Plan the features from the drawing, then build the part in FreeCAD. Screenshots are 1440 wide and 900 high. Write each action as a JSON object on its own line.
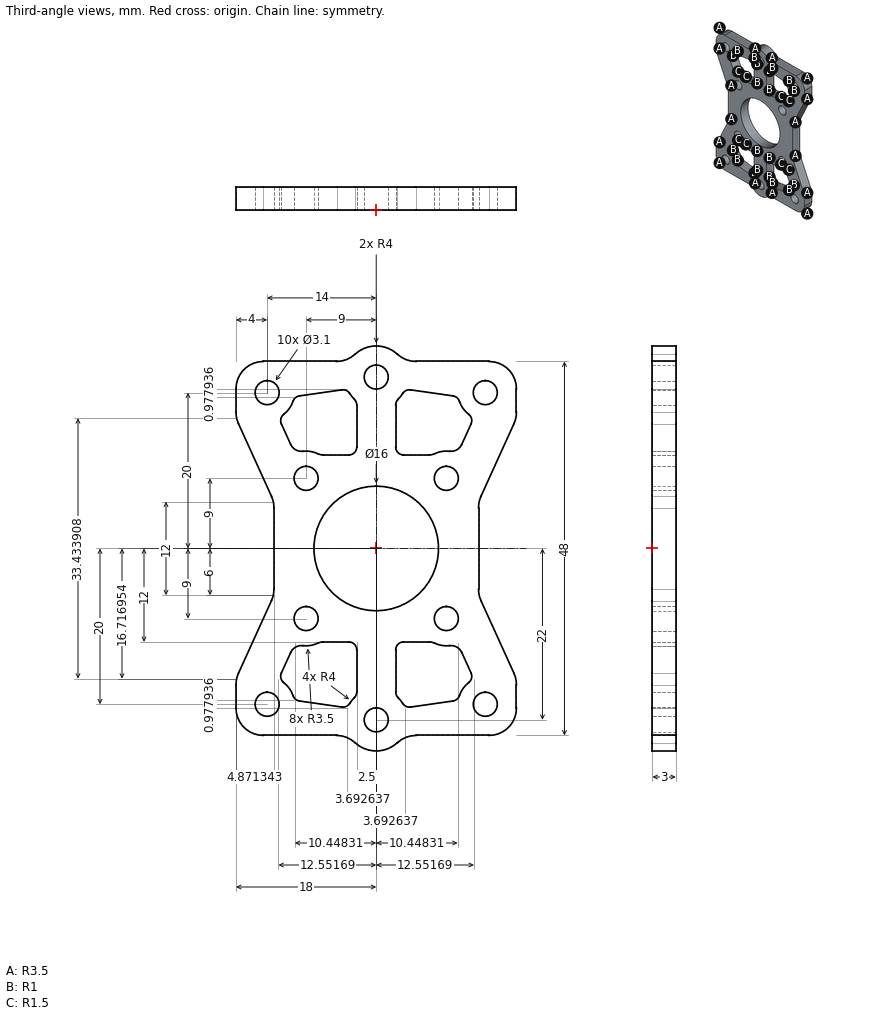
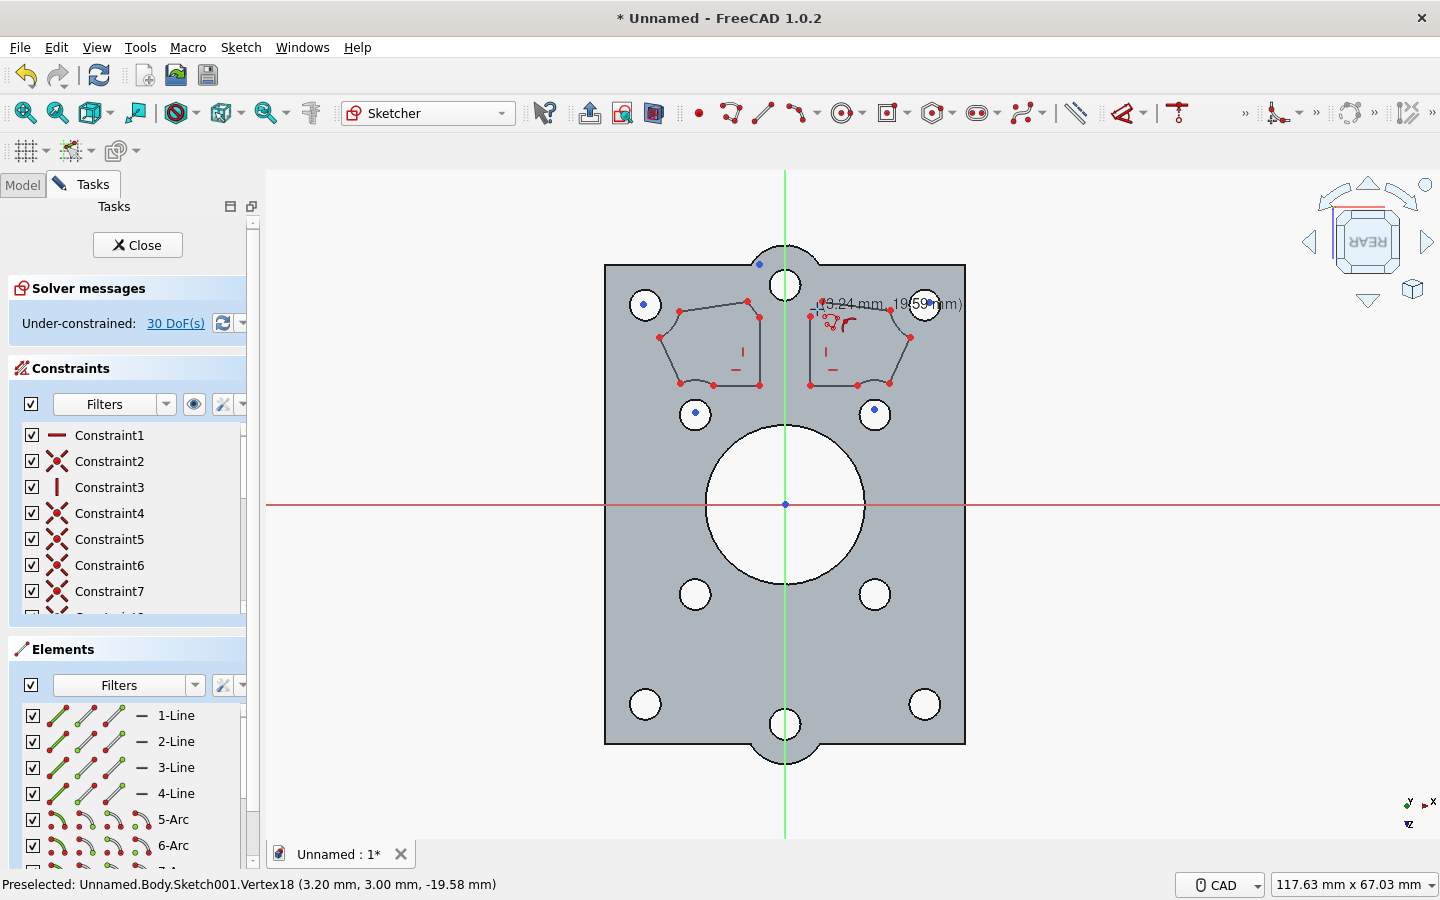
{"action": "left_click", "coordinate": [654, 445]}
{"action": "left_click", "coordinate": [605, 338]}
{"action": "left_click", "coordinate": [605, 672]}
{"action": "left_click", "coordinate": [654, 565]}
{"action": "left_click", "coordinate": [654, 446]}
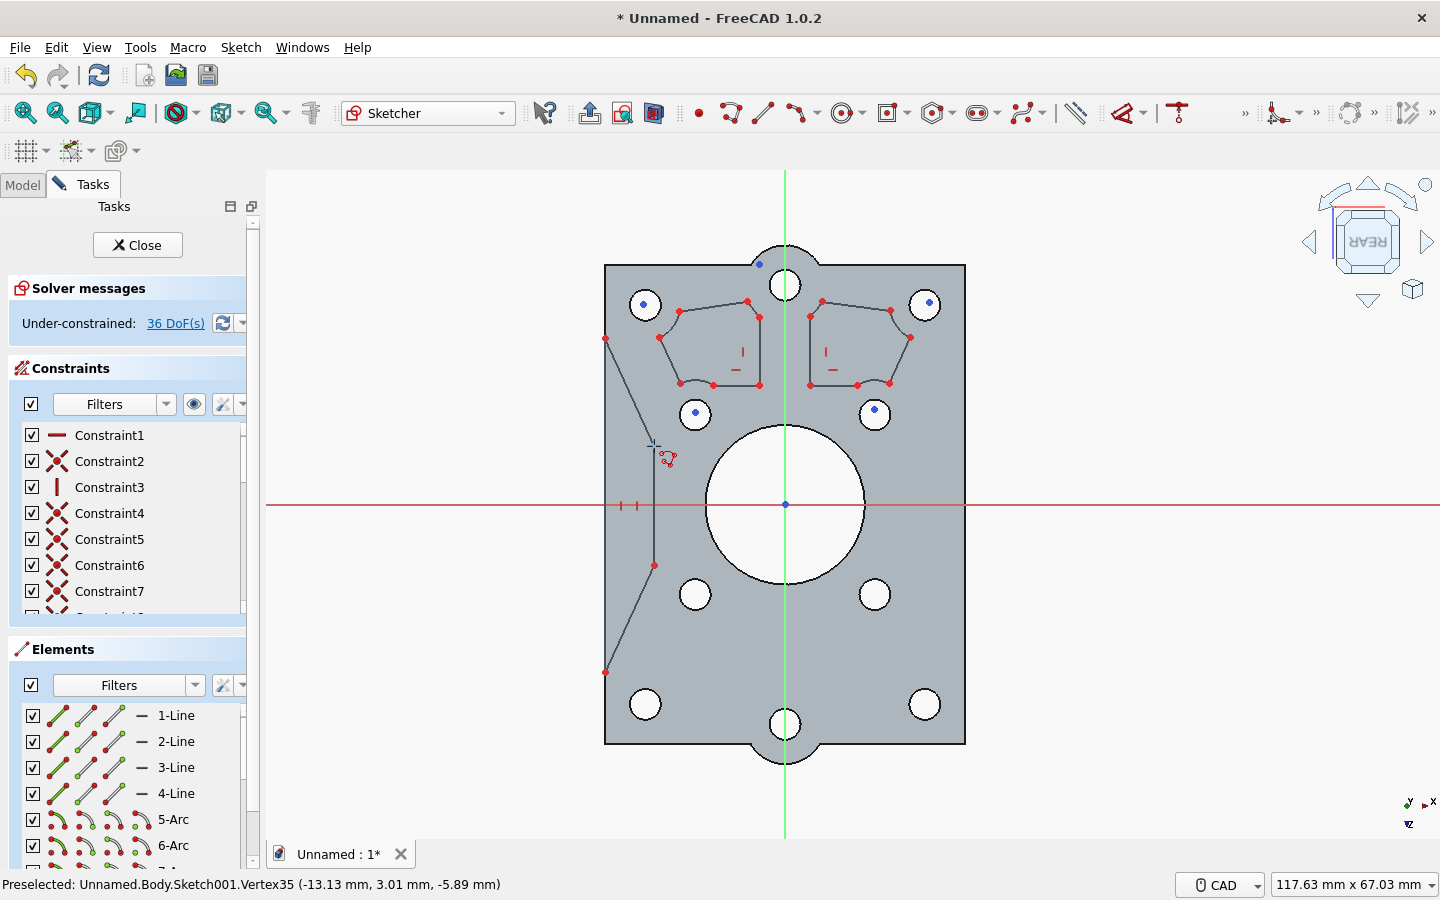
{"action": "left_click", "coordinate": [916, 445]}
{"action": "left_click", "coordinate": [916, 565]}
{"action": "left_click", "coordinate": [965, 672]}
{"action": "left_click", "coordinate": [965, 338]}
{"action": "left_click", "coordinate": [916, 446]}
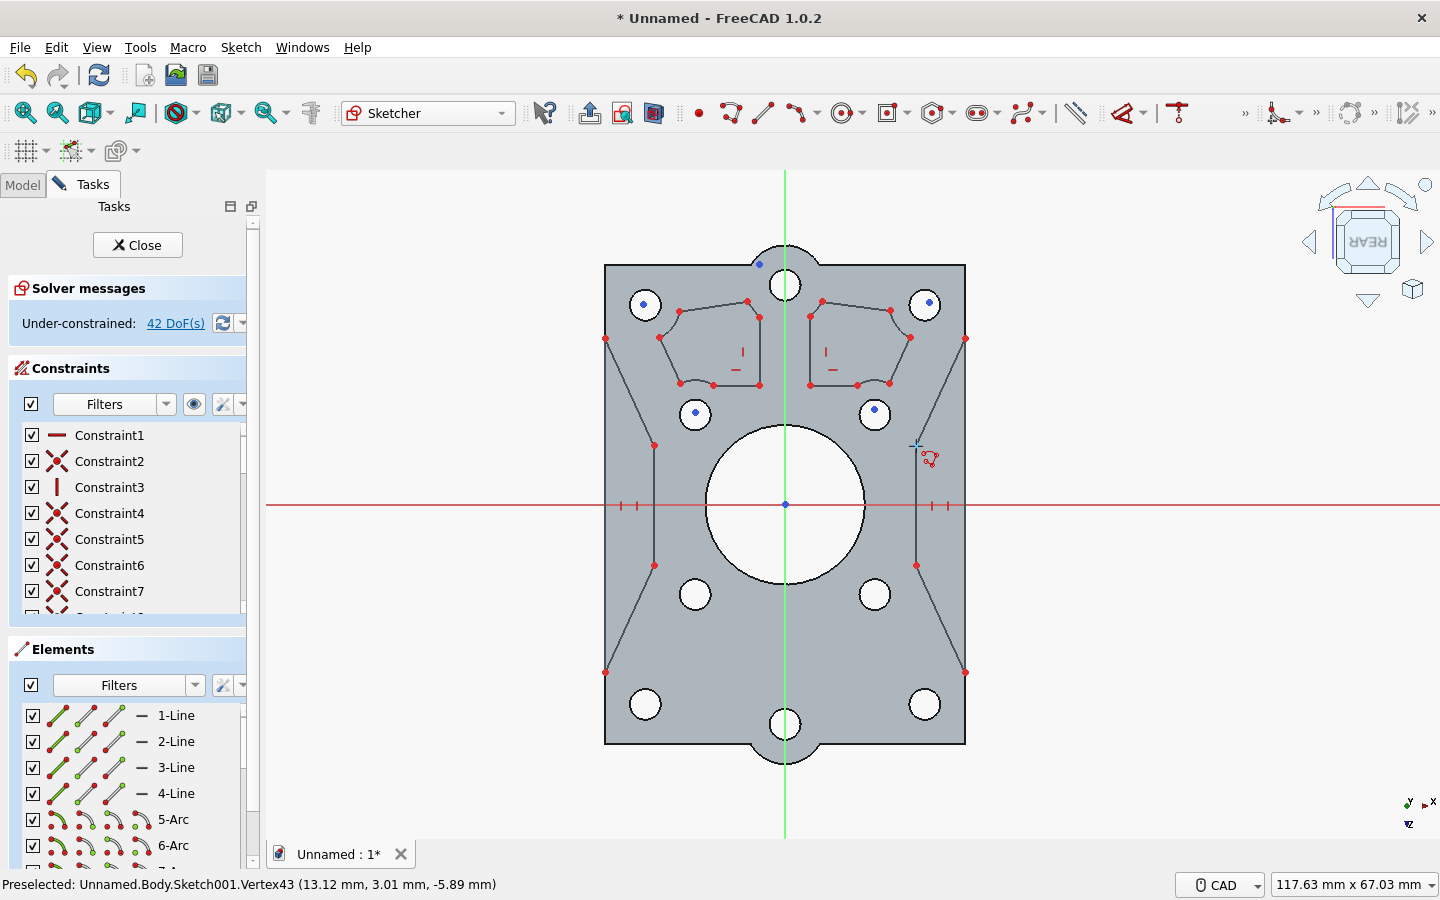
{"action": "key", "text": "g l"}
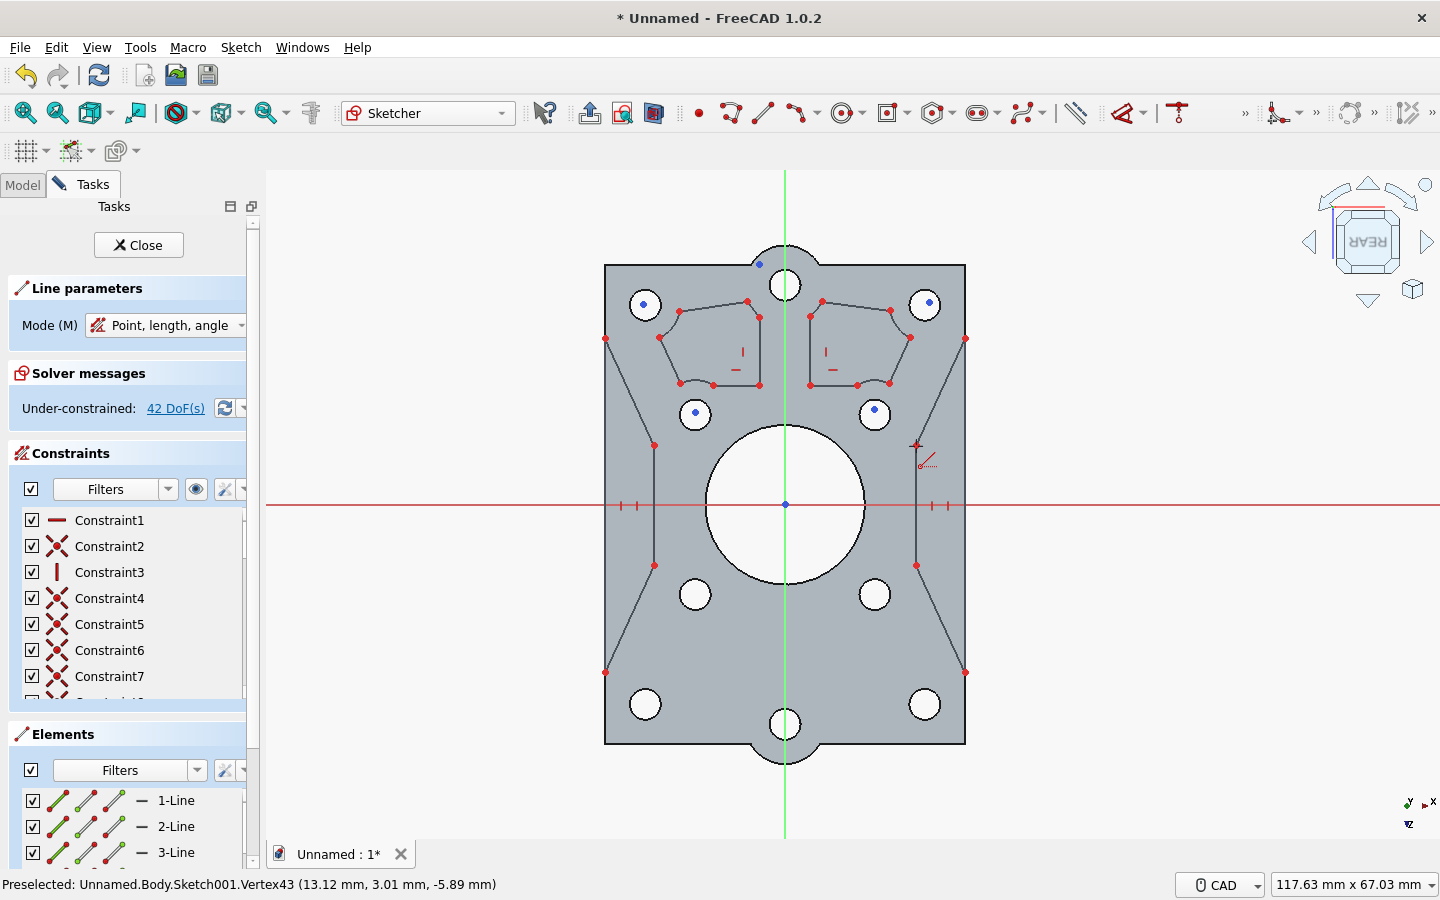
{"action": "left_click", "coordinate": [680, 699]}
{"action": "left_click", "coordinate": [748, 709]}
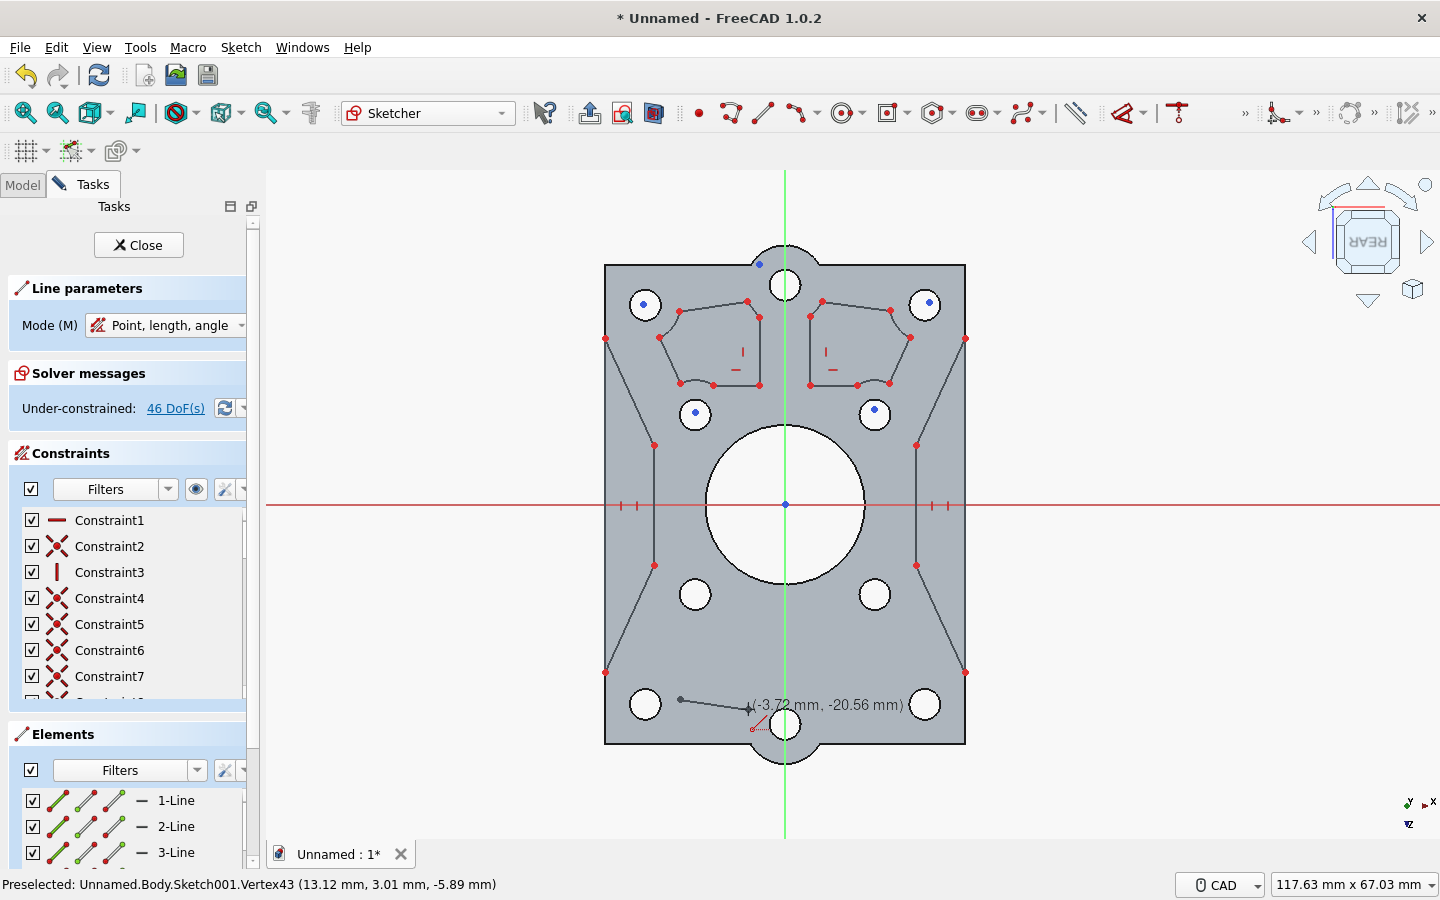
{"action": "left_click", "coordinate": [732, 114]}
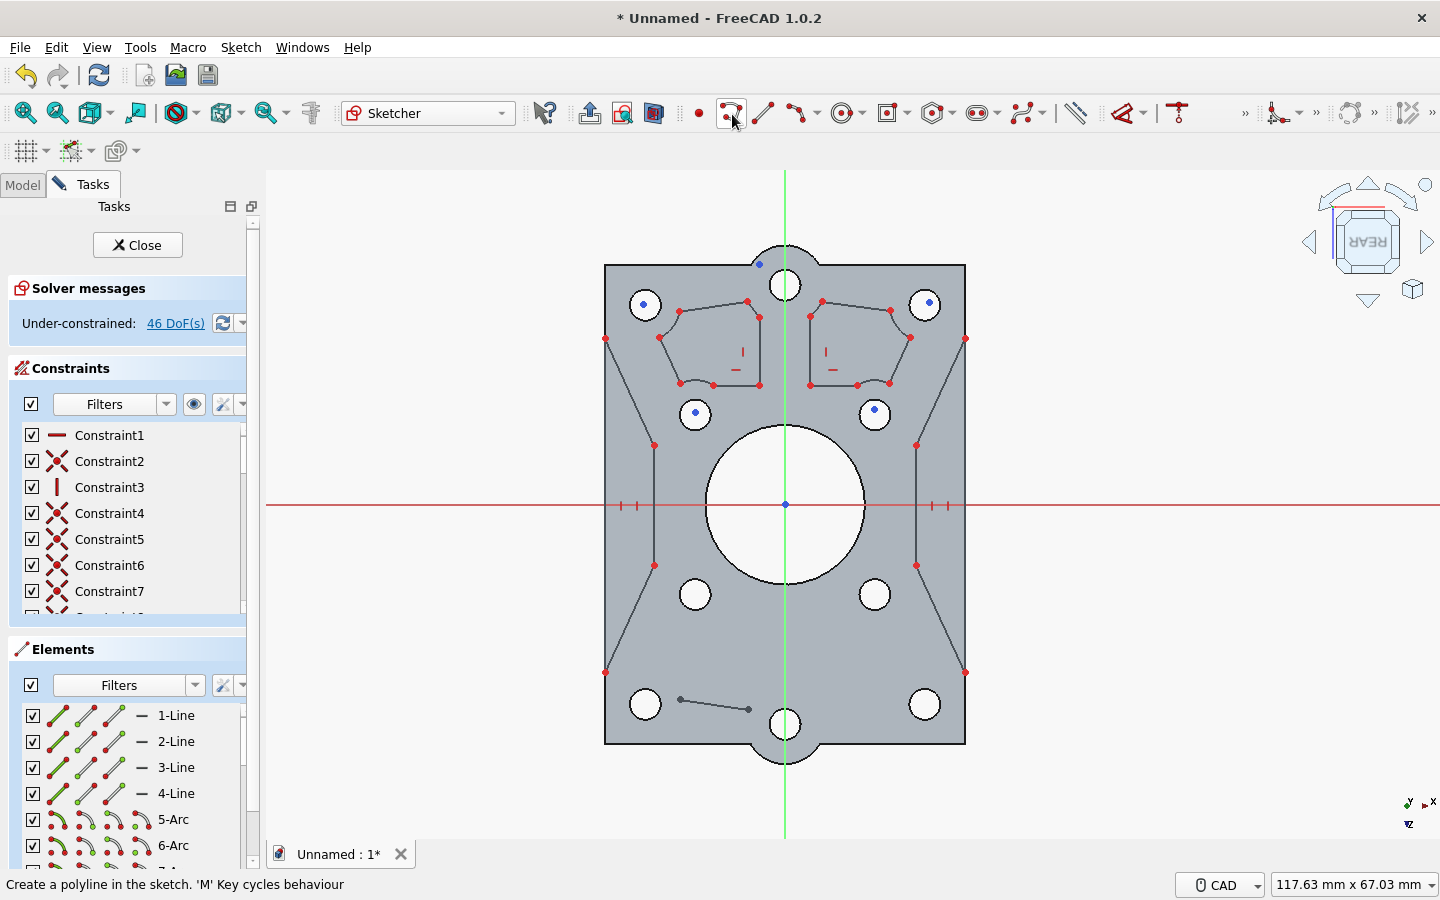
{"action": "left_click", "coordinate": [760, 693]}
{"action": "left_click", "coordinate": [760, 625]}
{"action": "left_click", "coordinate": [713, 625]}
{"action": "right_click", "coordinate": [713, 625]}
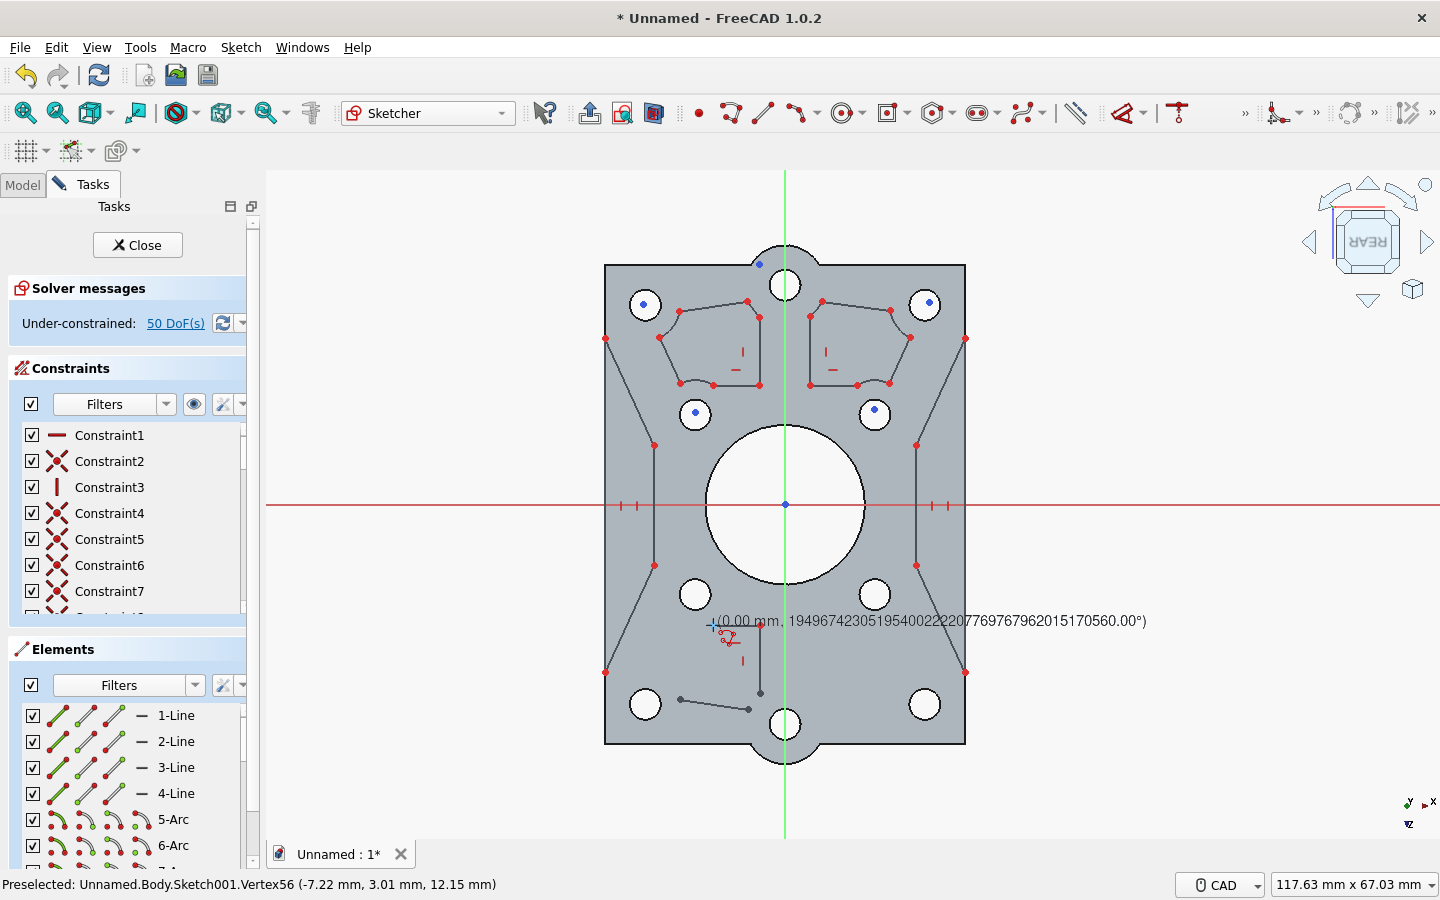
{"action": "left_click", "coordinate": [764, 114]}